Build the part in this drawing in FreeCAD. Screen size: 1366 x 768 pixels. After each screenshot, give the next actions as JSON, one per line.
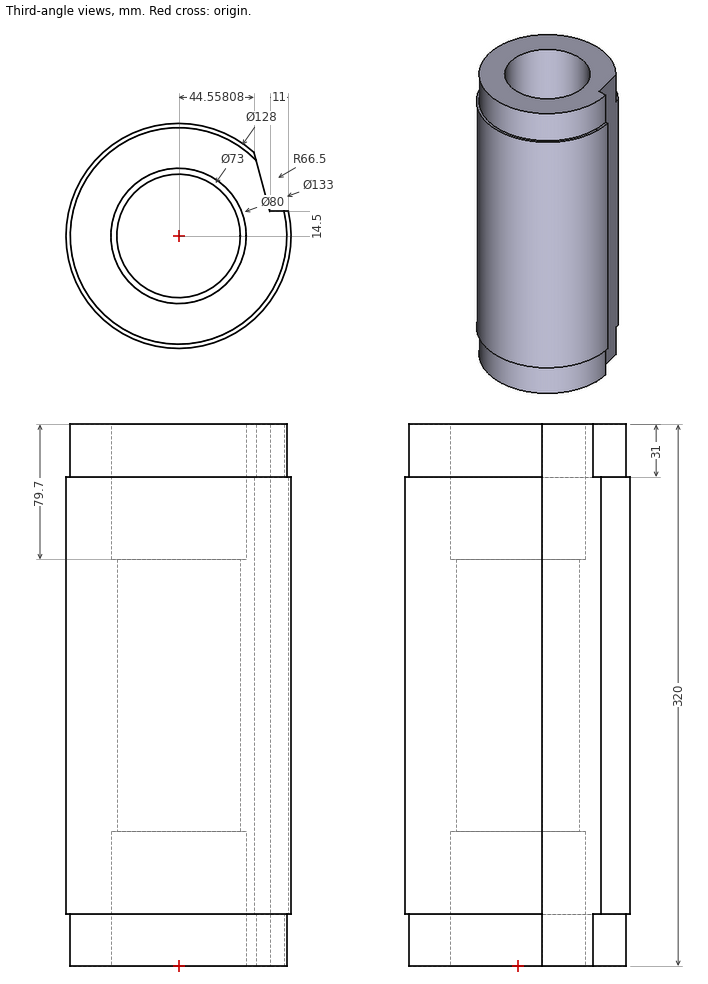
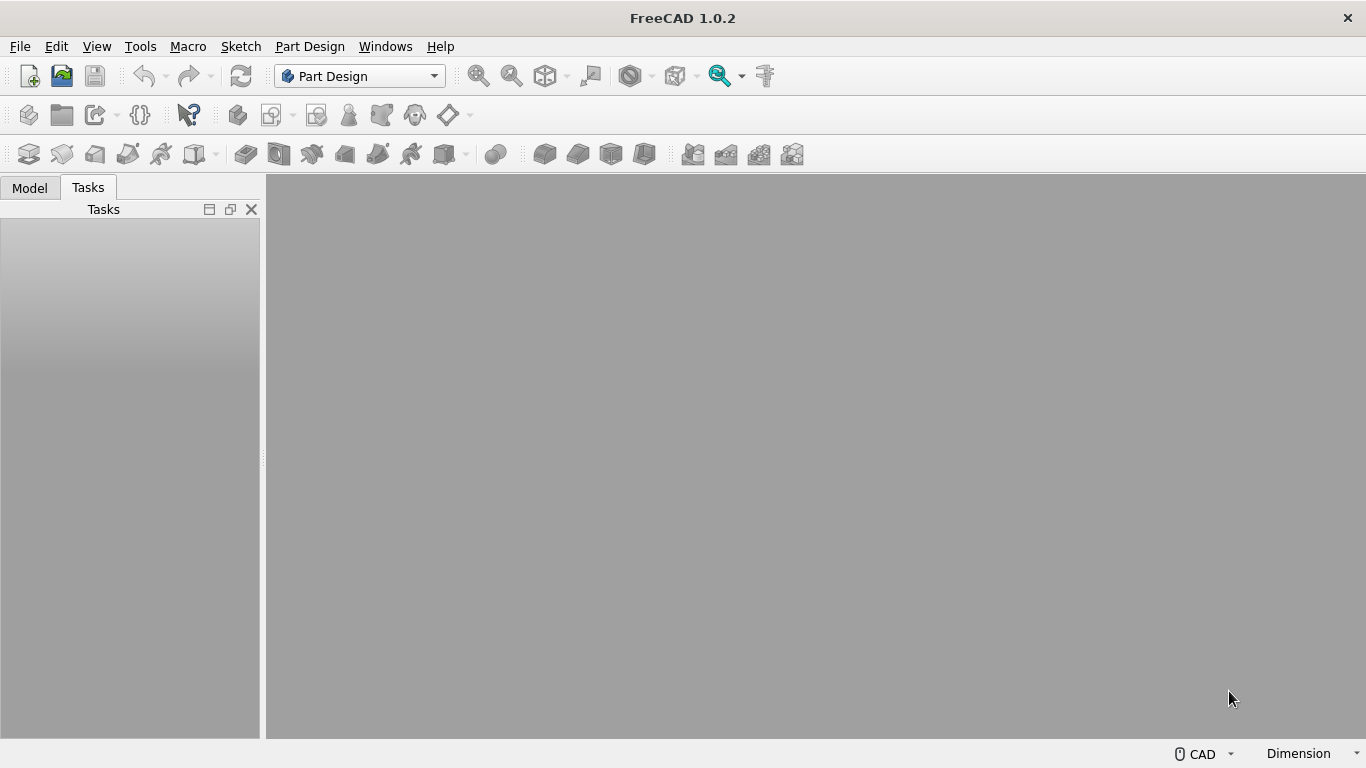
{"action": "key", "text": "ctrl+n"}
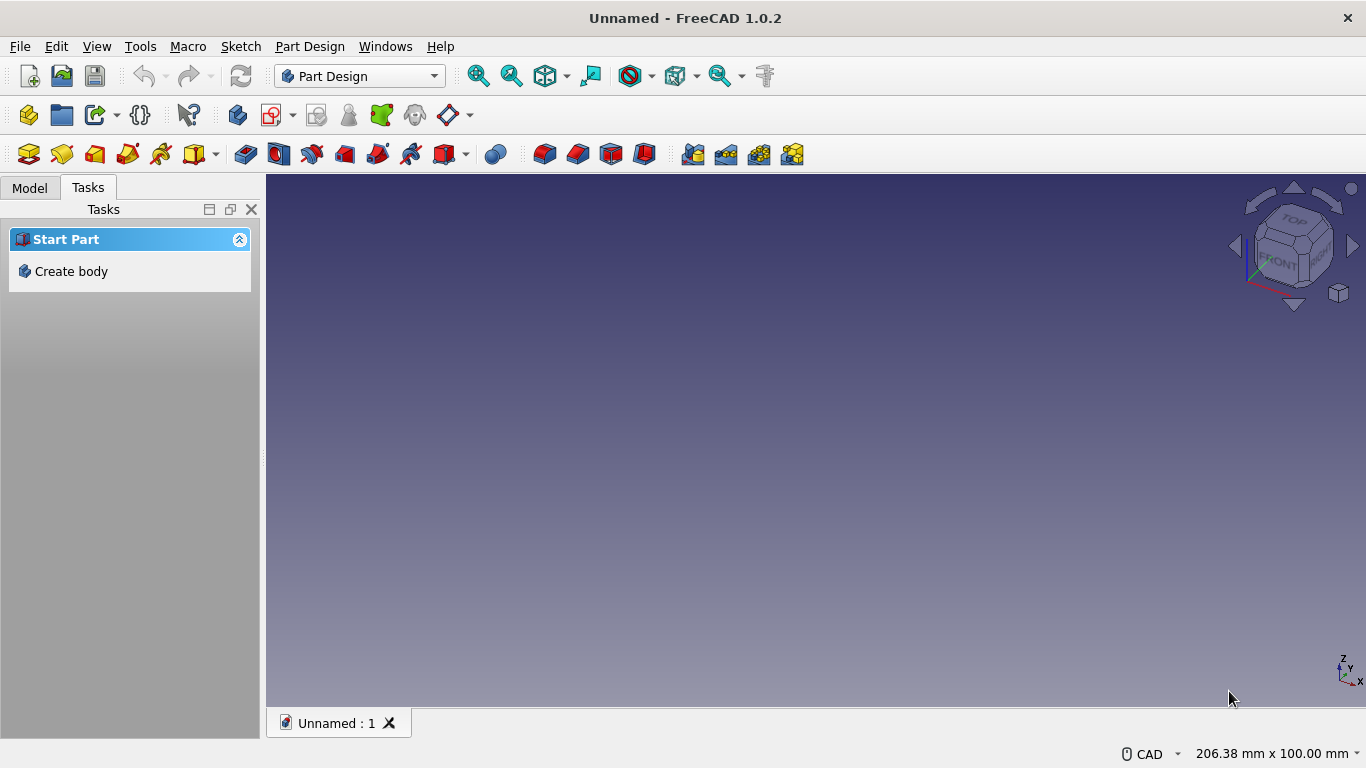
{"action": "left_click", "coordinate": [270, 116]}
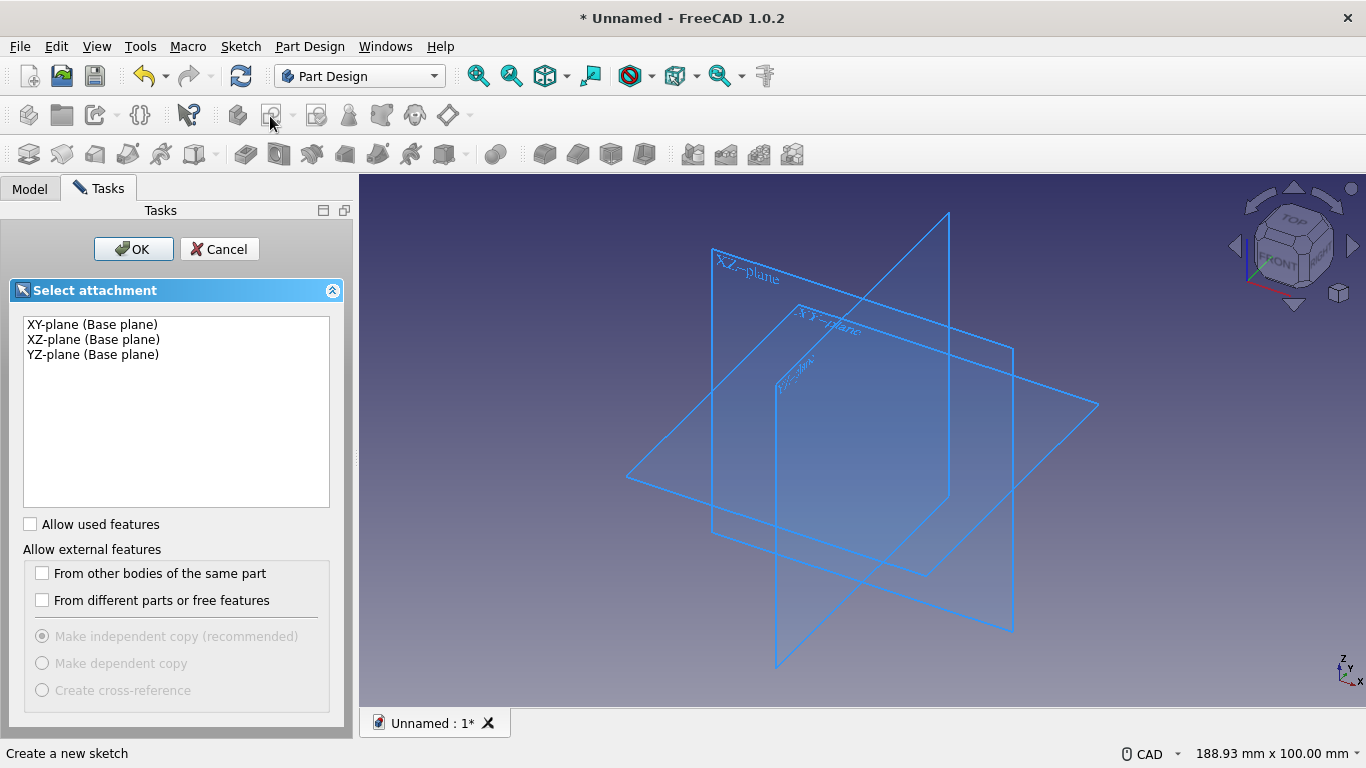
{"action": "left_click", "coordinate": [84, 324]}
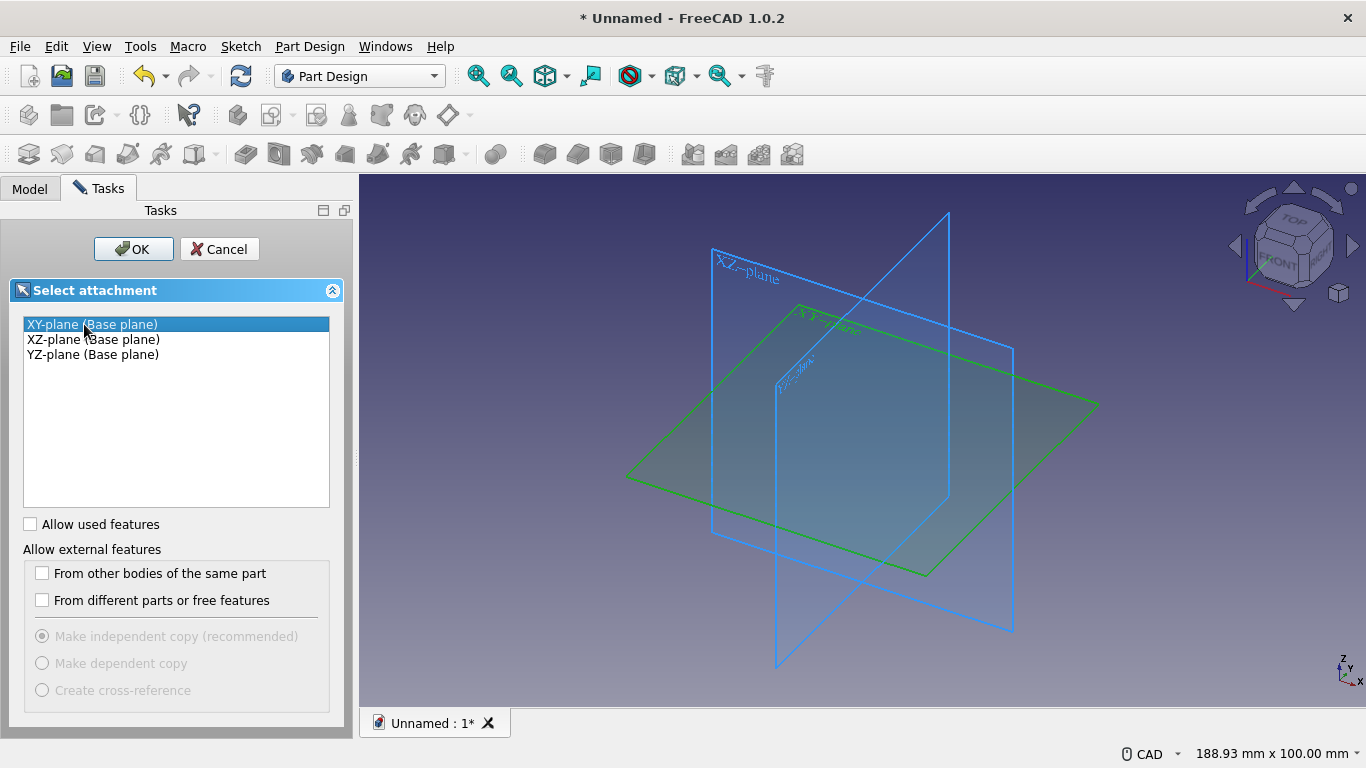
{"action": "left_click", "coordinate": [134, 249]}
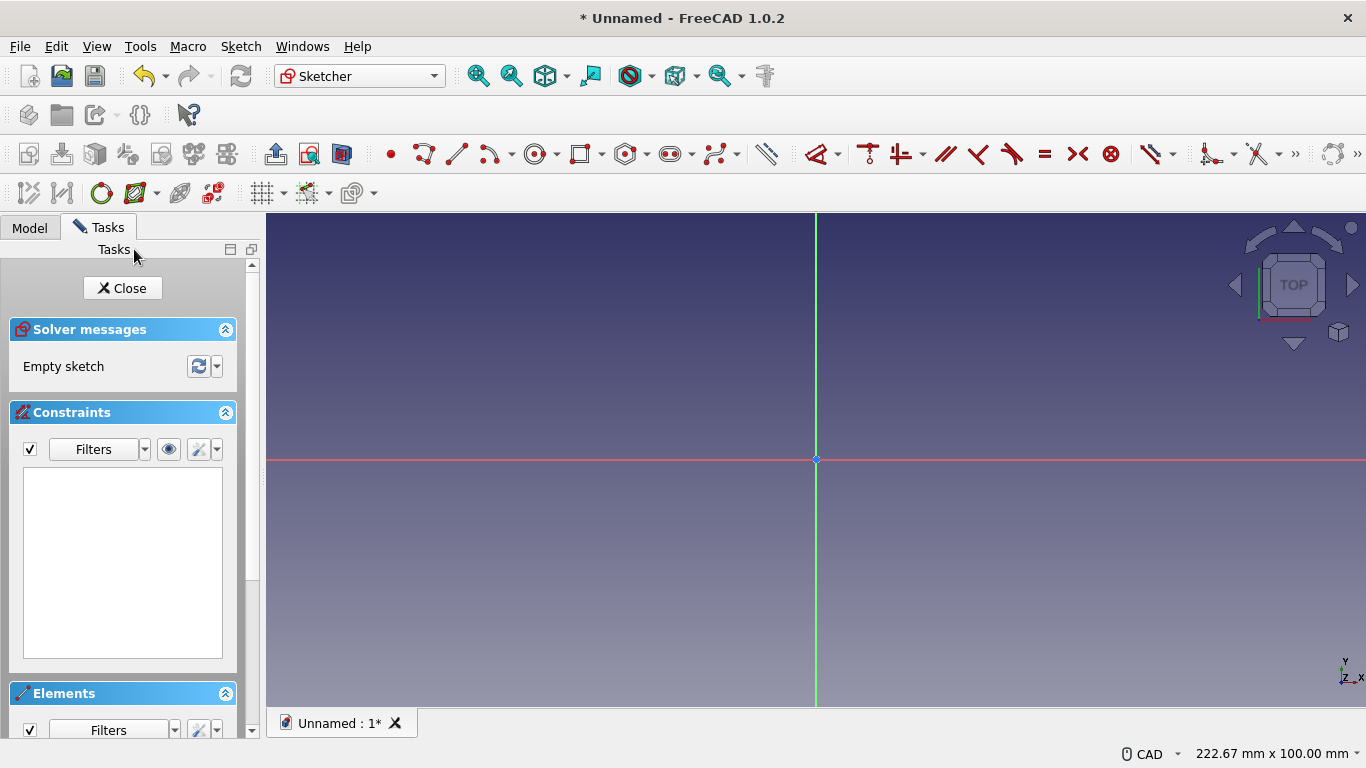
{"action": "scroll", "coordinate": [692, 460], "scroll_direction": "down", "scroll_amount": 4}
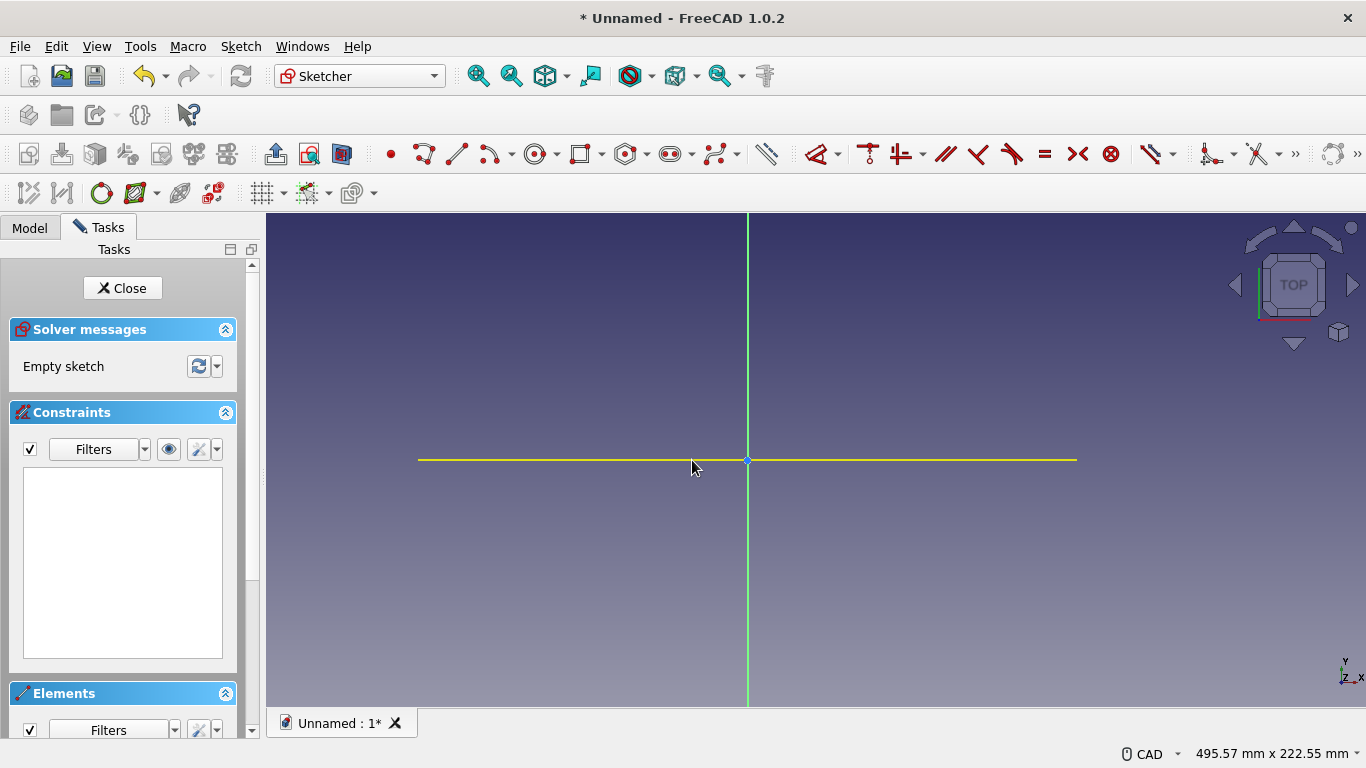
{"action": "left_click", "coordinate": [534, 154]}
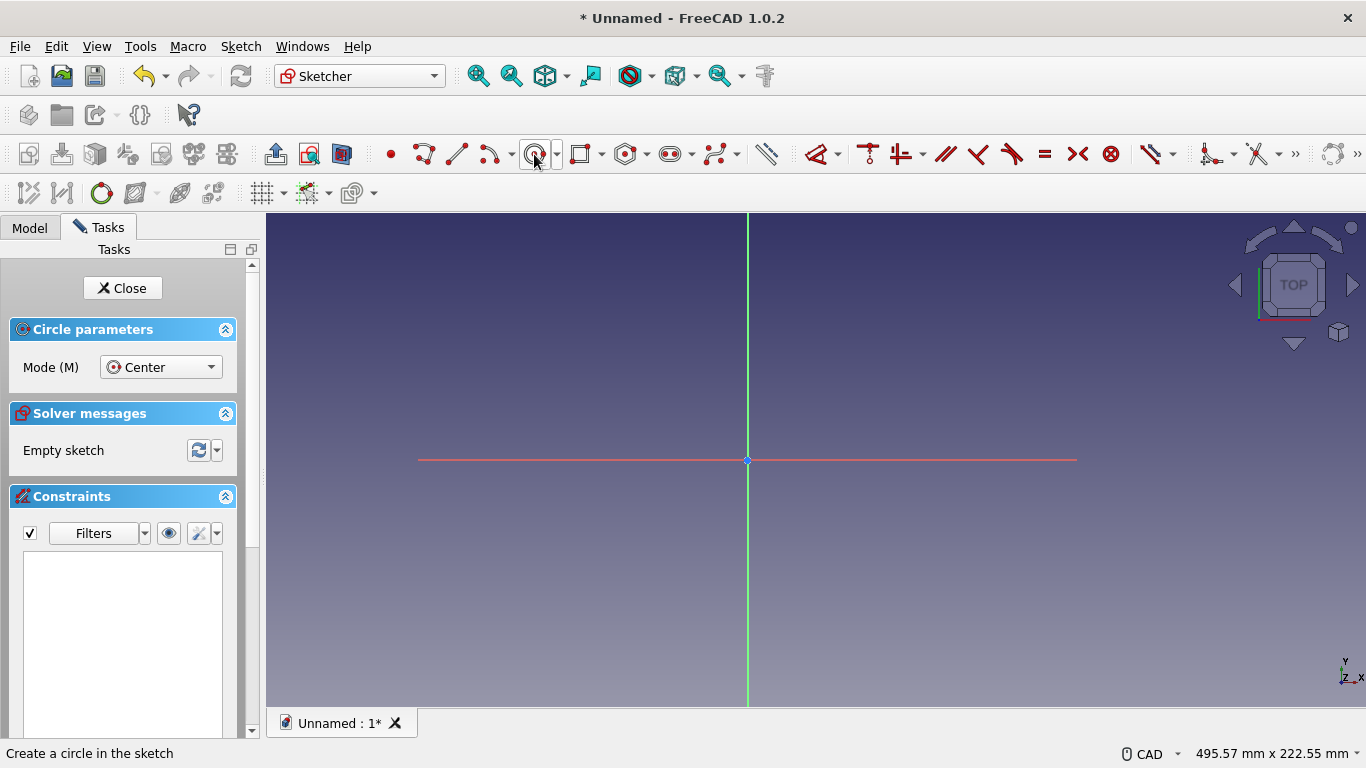
{"action": "left_click", "coordinate": [748, 460]}
{"action": "mouse_move", "coordinate": [852, 356]}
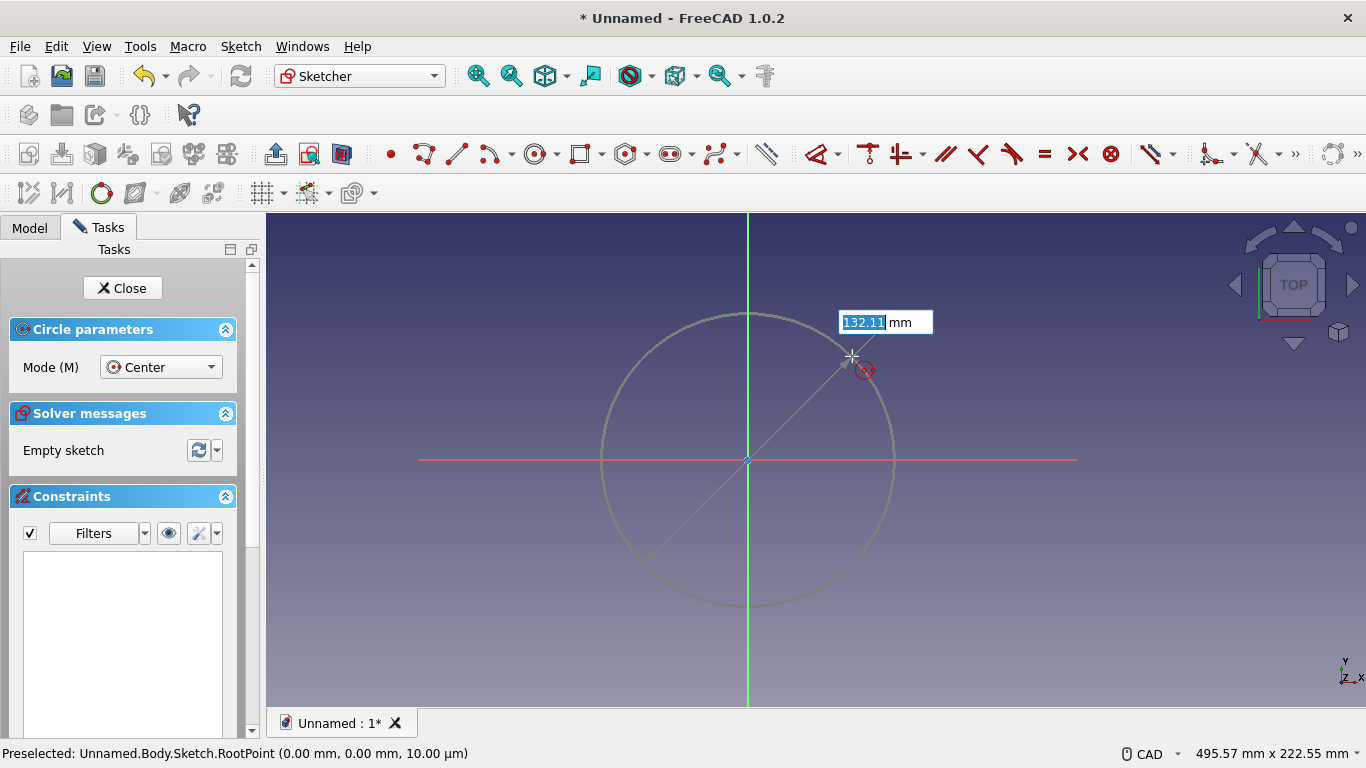
{"action": "type", "text": "133"}
{"action": "key", "text": "Return"}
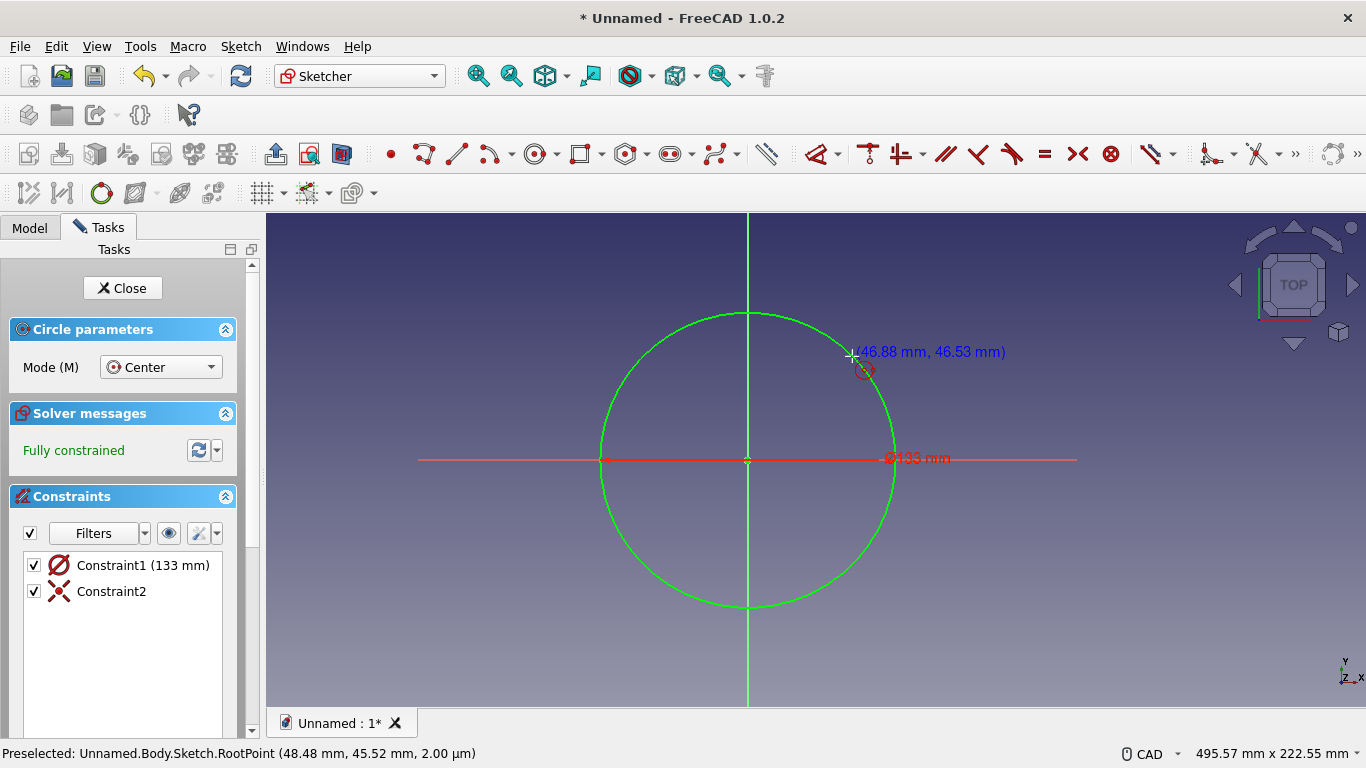
{"action": "left_click", "coordinate": [748, 460]}
{"action": "mouse_move", "coordinate": [805, 403]}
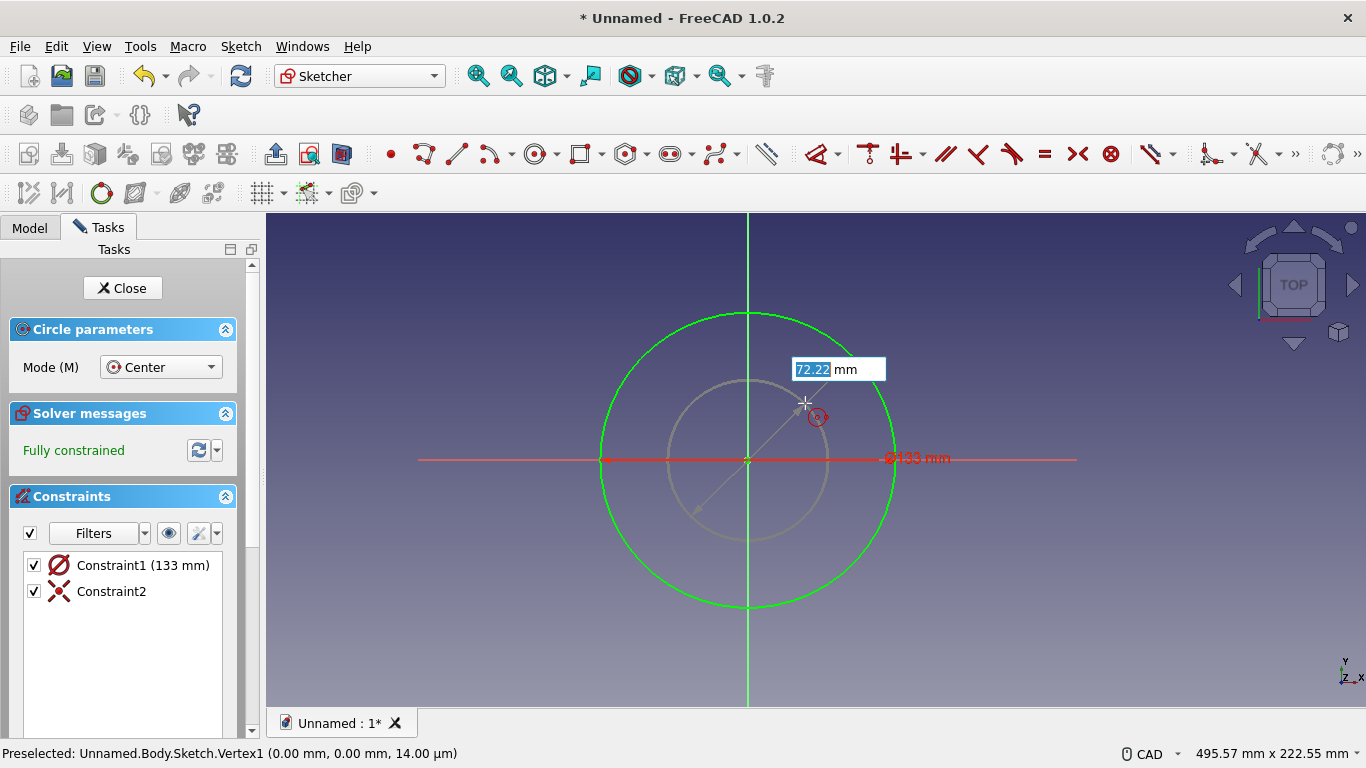
{"action": "type", "text": "73"}
{"action": "key", "text": "Return"}
{"action": "key", "text": "Escape"}